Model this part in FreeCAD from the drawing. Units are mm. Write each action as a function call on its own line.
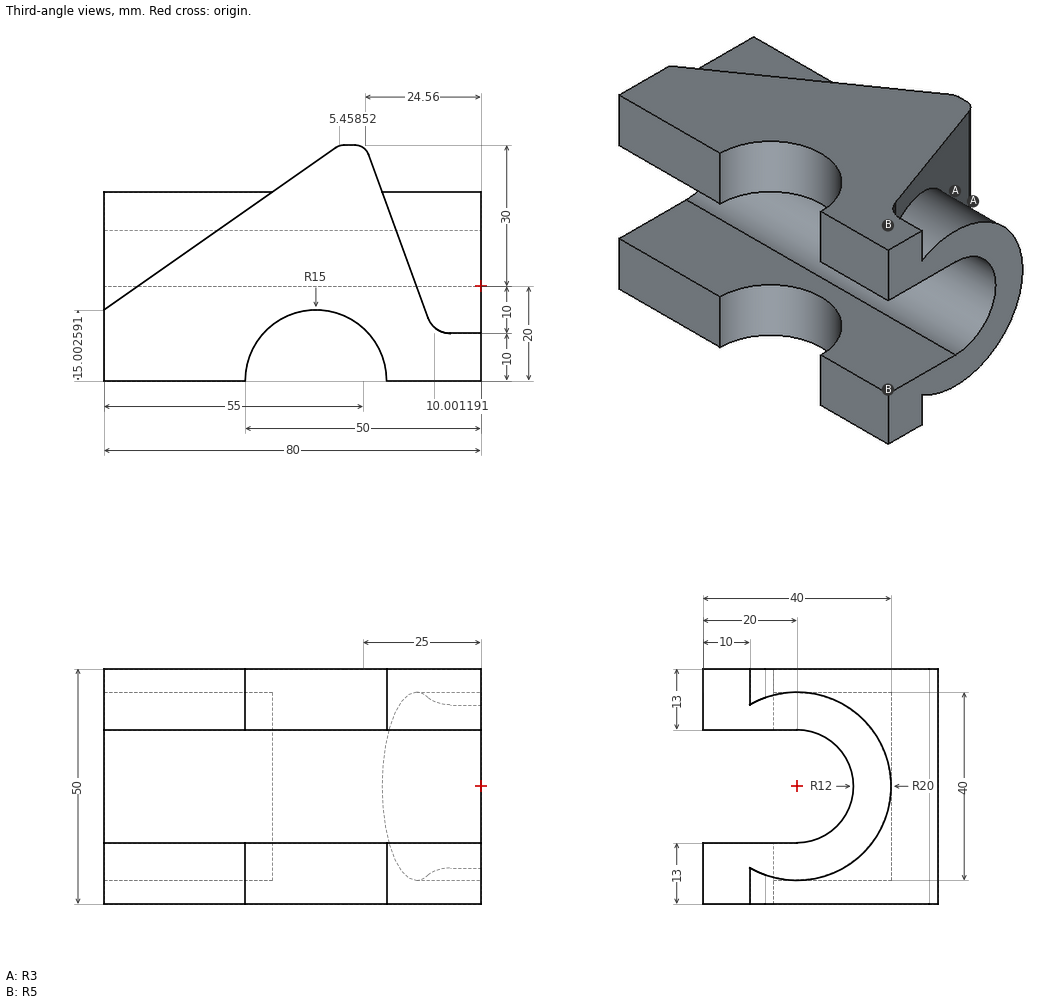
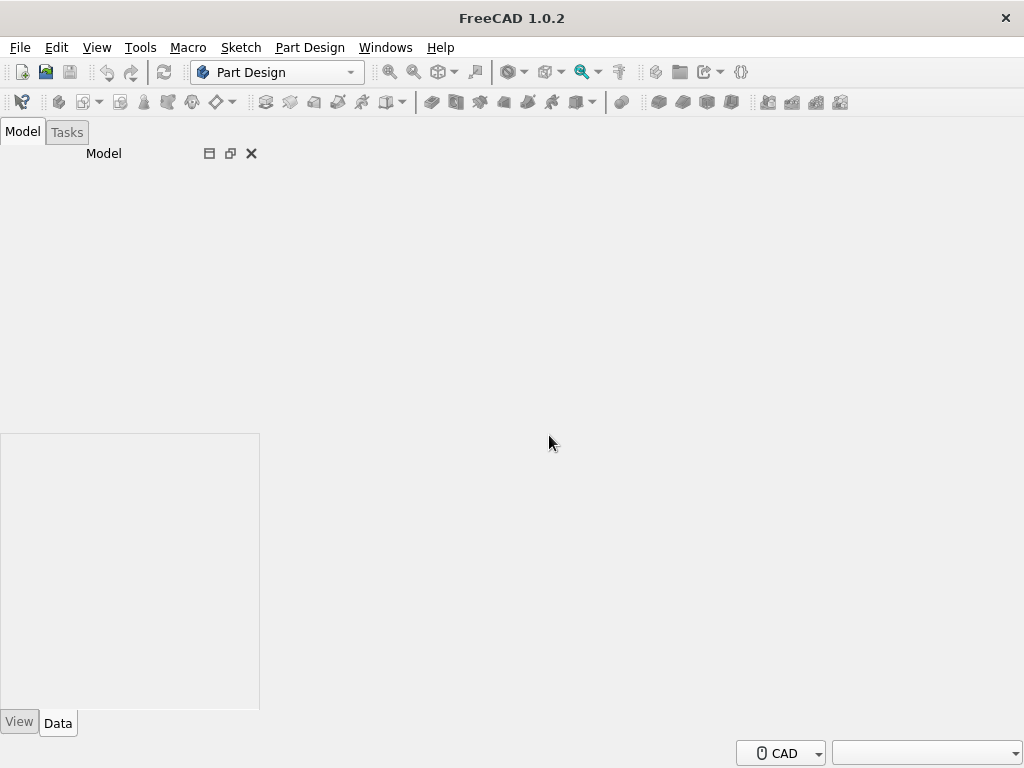
click(22, 72)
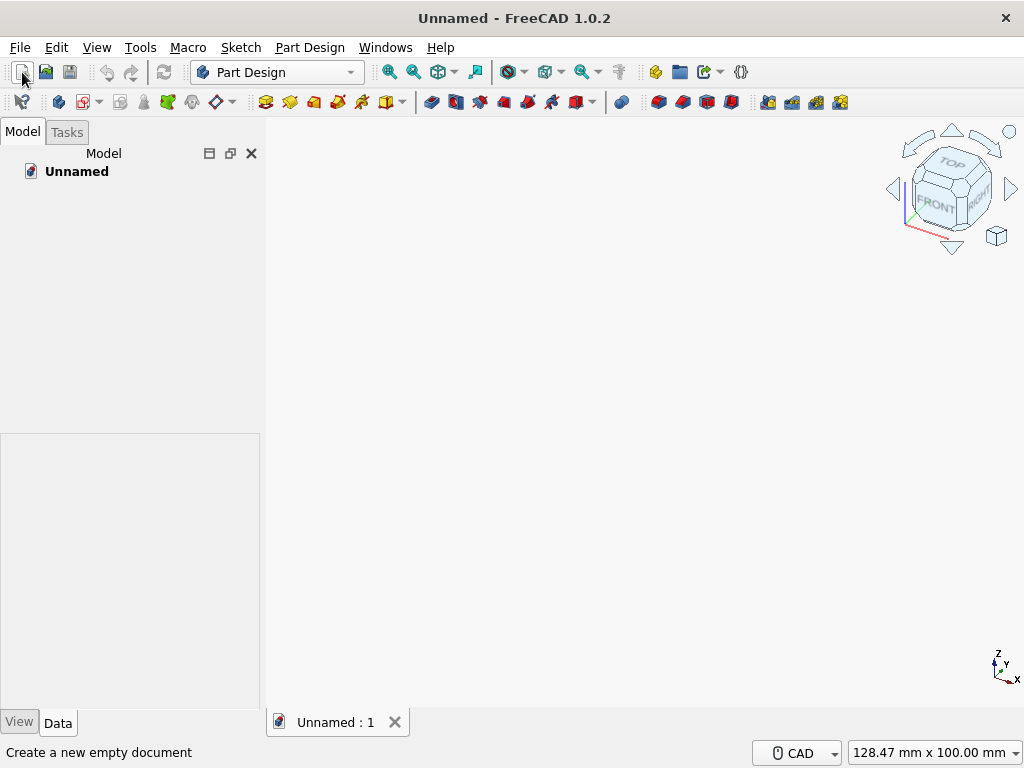
click(84, 102)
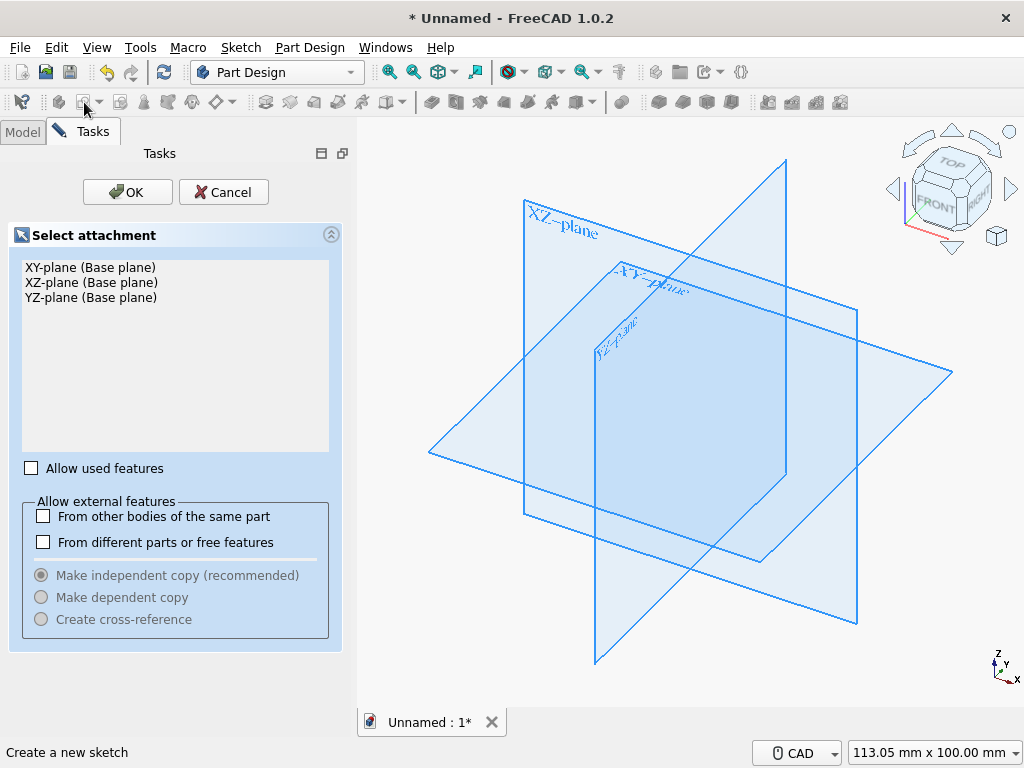
click(82, 298)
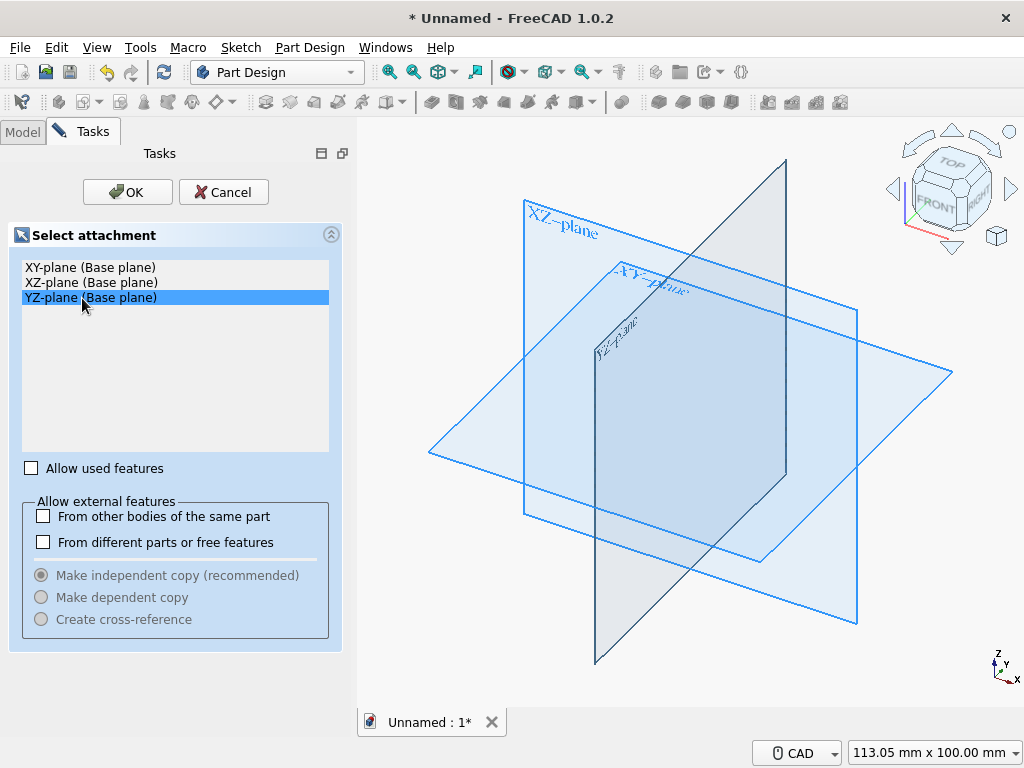
click(128, 192)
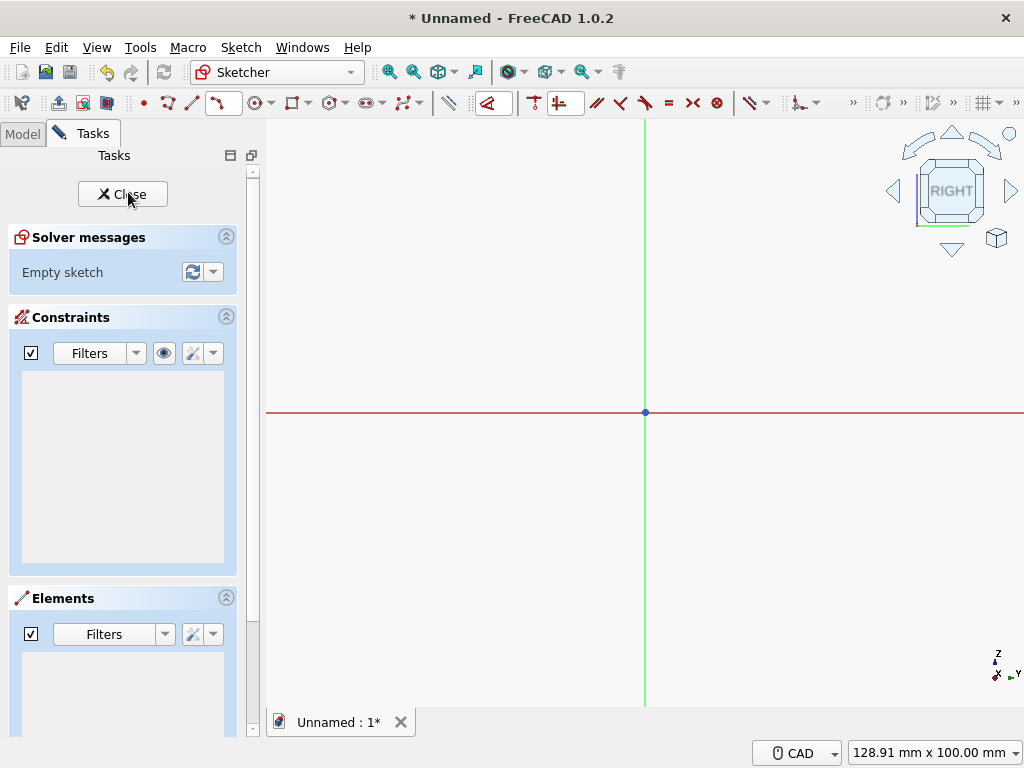
key(g)
key(m)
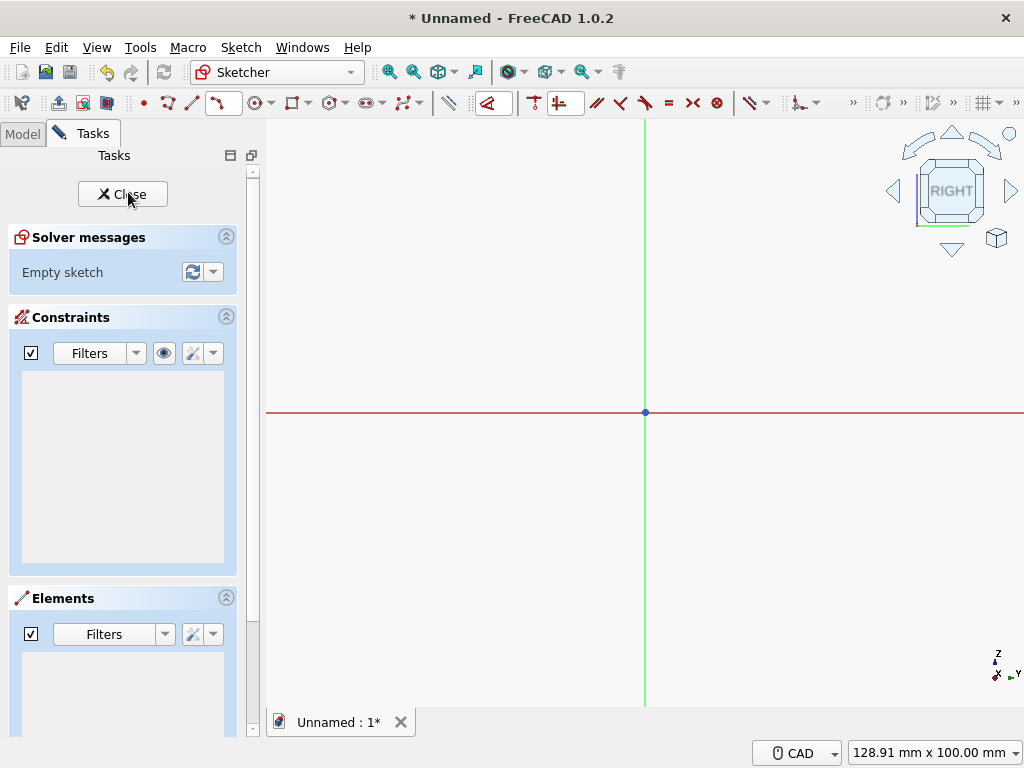
click(586, 311)
click(586, 266)
click(527, 266)
click(527, 342)
click(645, 342)
right_click(645, 342)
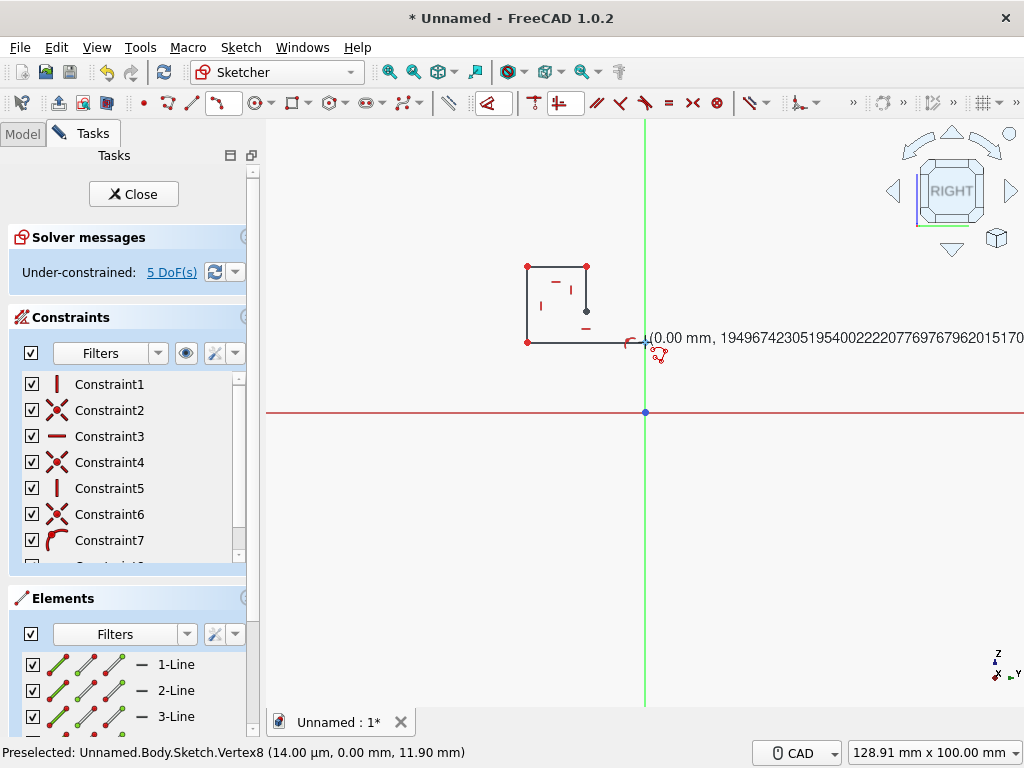
click(645, 484)
click(527, 484)
click(527, 560)
click(586, 560)
click(586, 515)
right_click(586, 515)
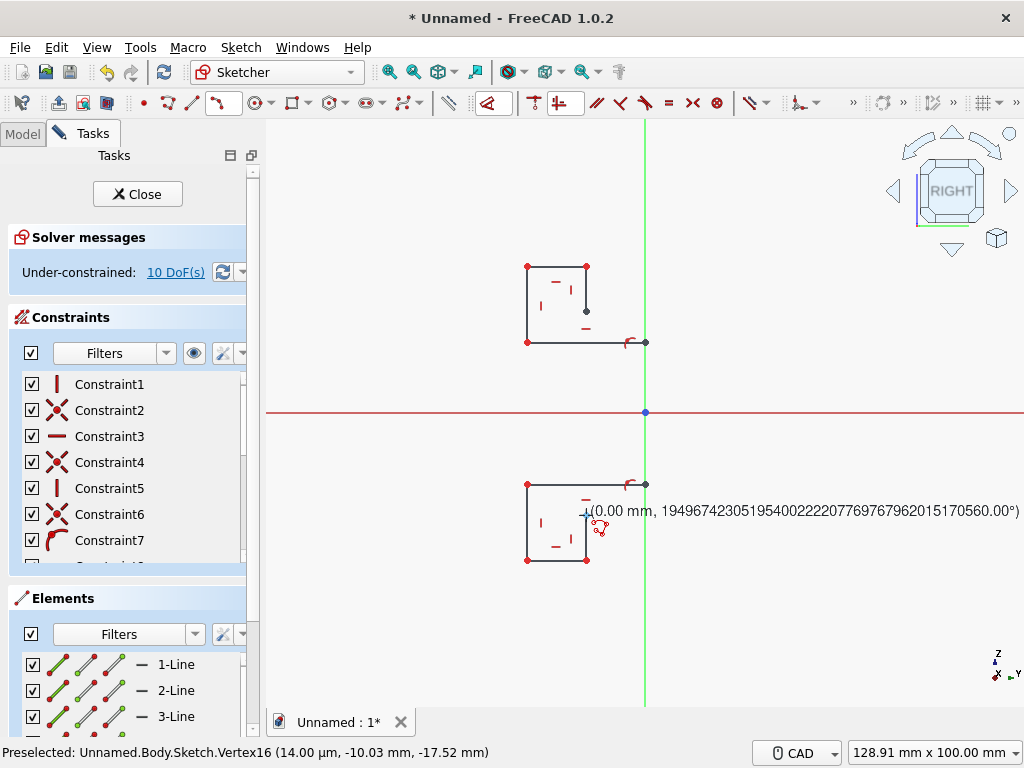
click(218, 104)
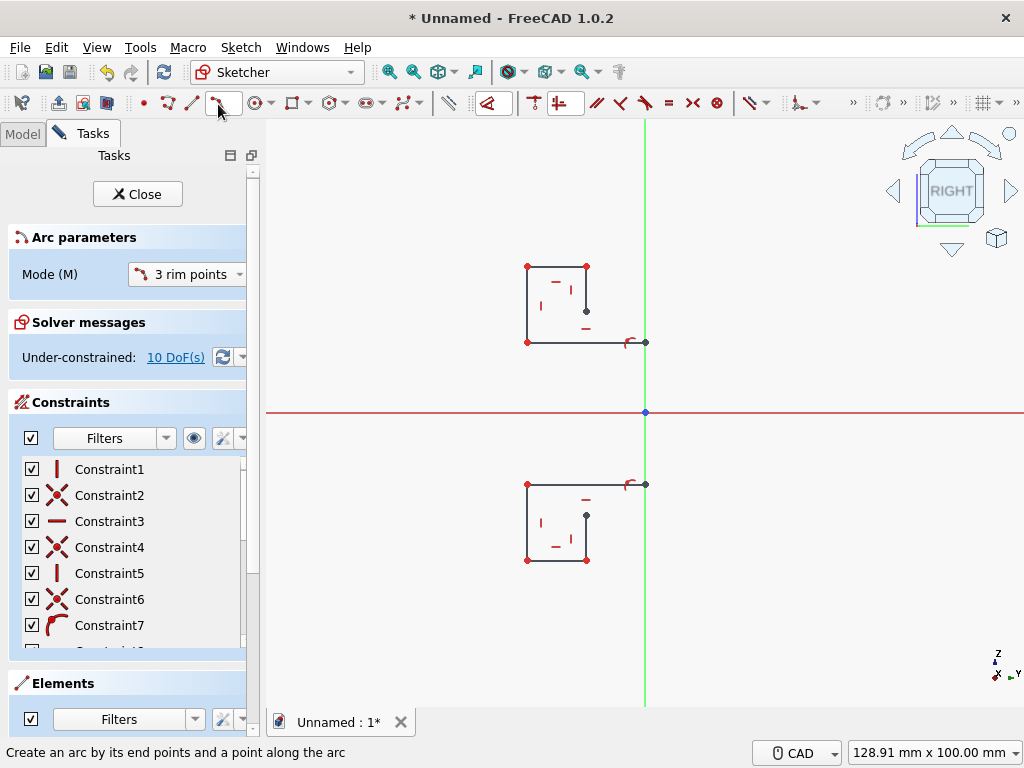
click(645, 343)
click(645, 485)
click(712, 435)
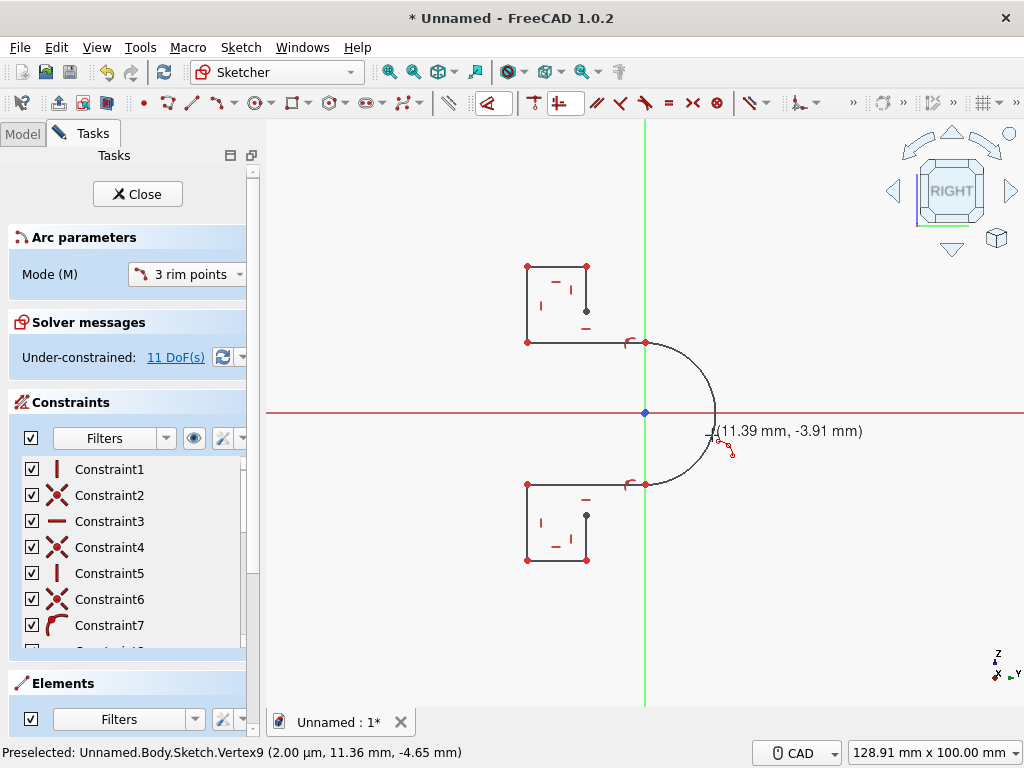
click(586, 516)
click(586, 312)
click(752, 461)
key(Escape)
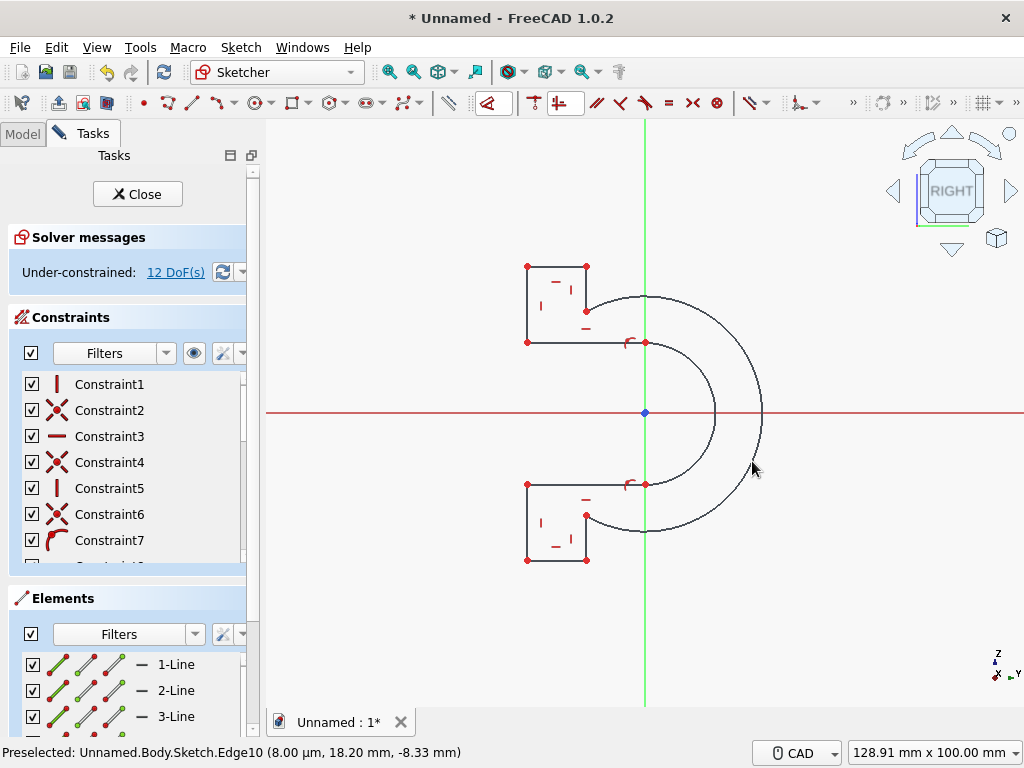
click(562, 343)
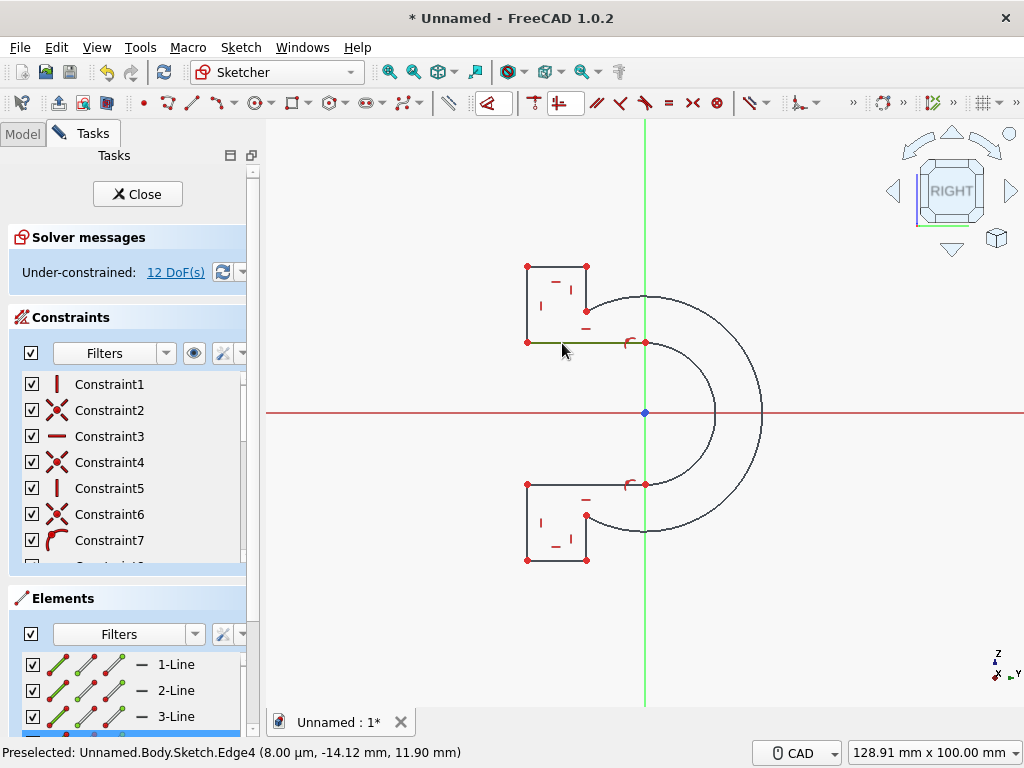
click(702, 456)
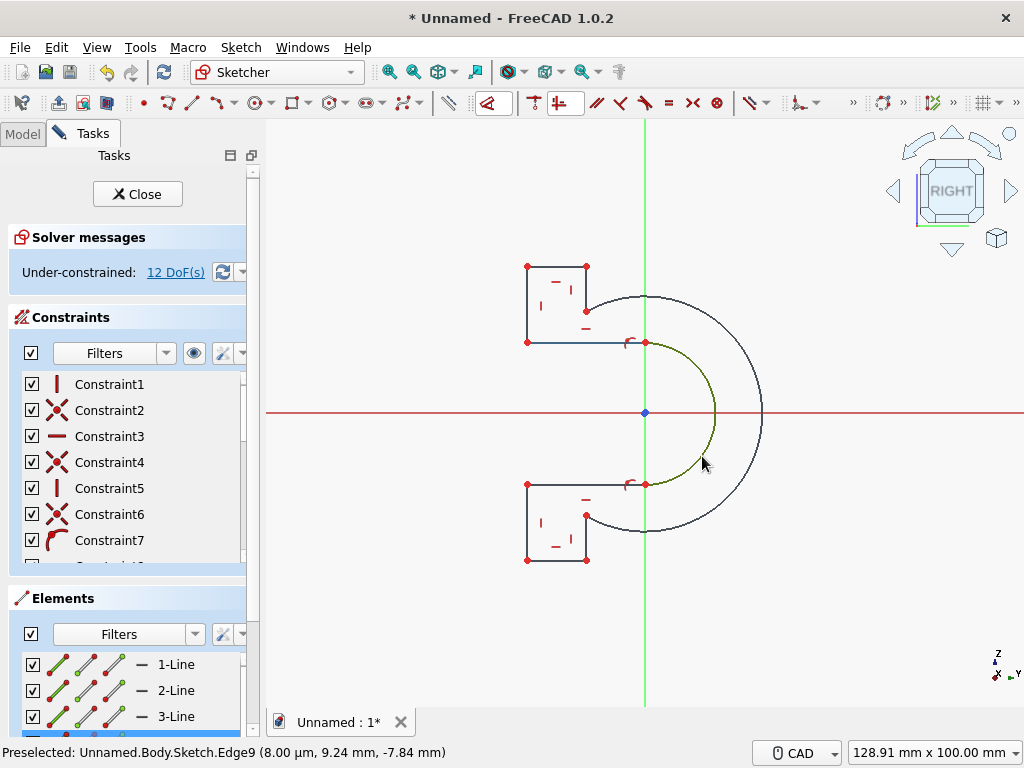
click(646, 104)